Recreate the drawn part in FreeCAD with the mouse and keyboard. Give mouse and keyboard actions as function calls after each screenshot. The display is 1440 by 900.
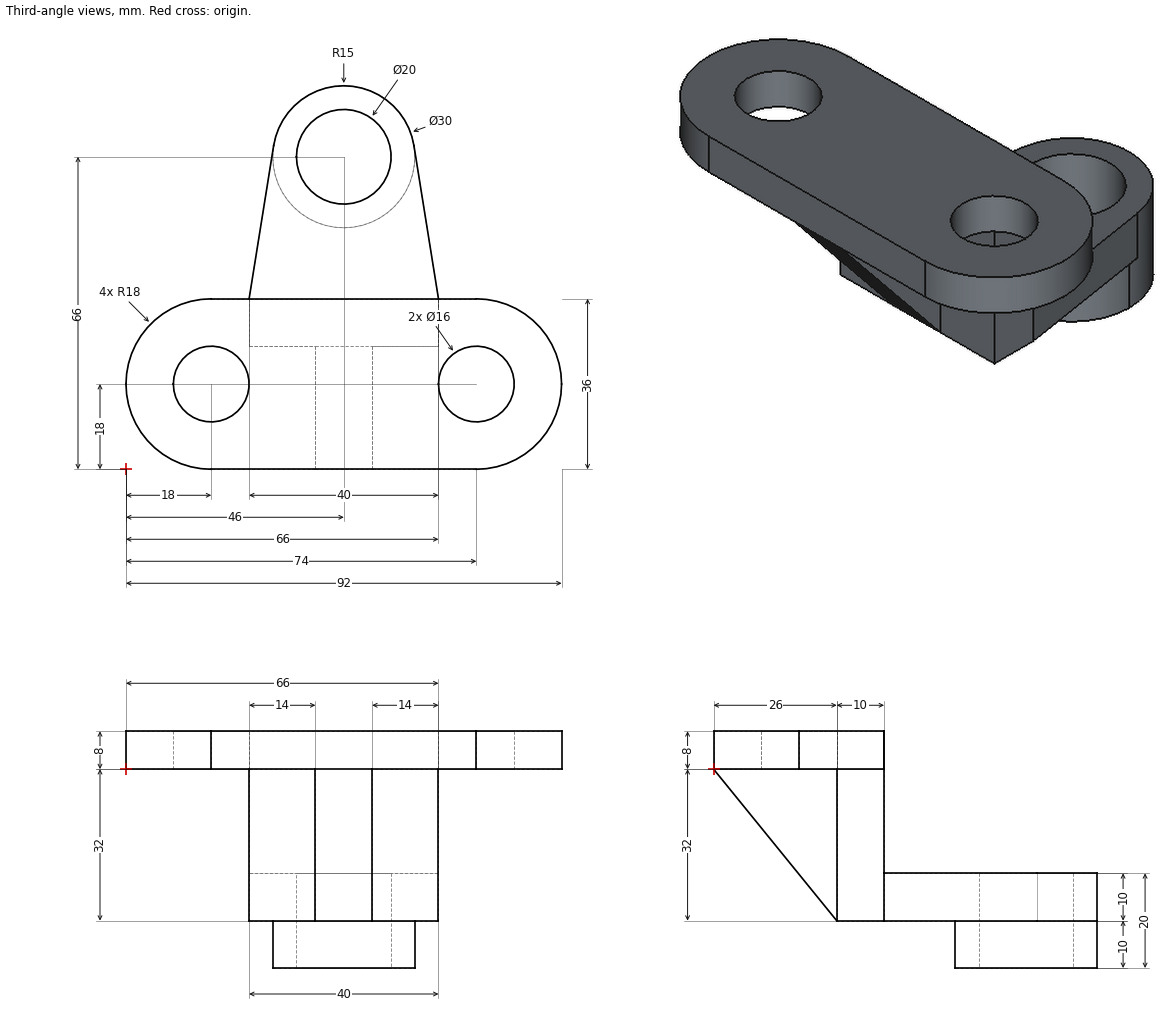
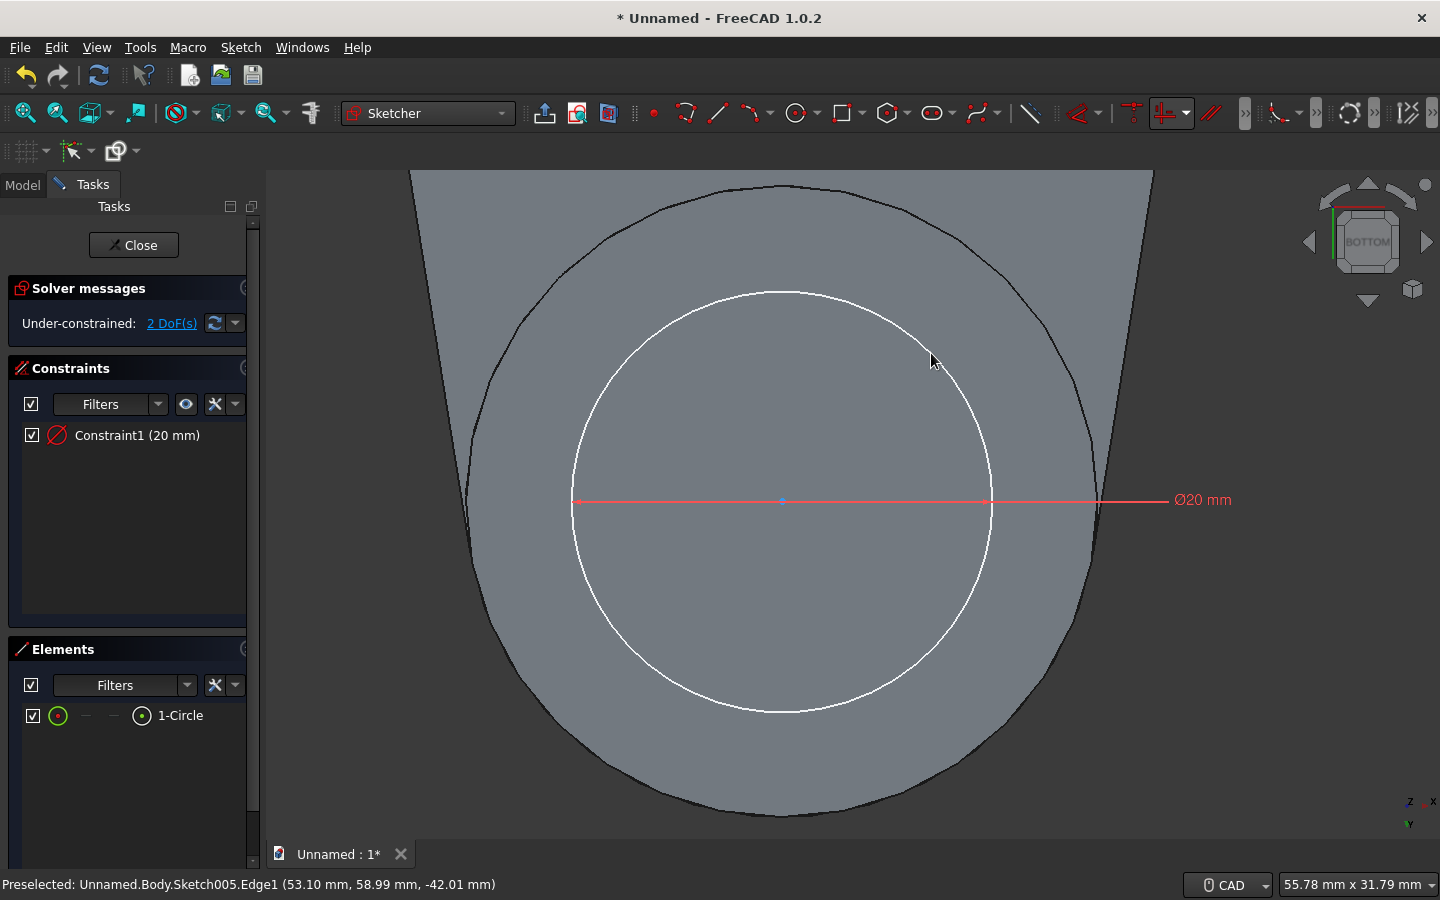
click(1078, 114)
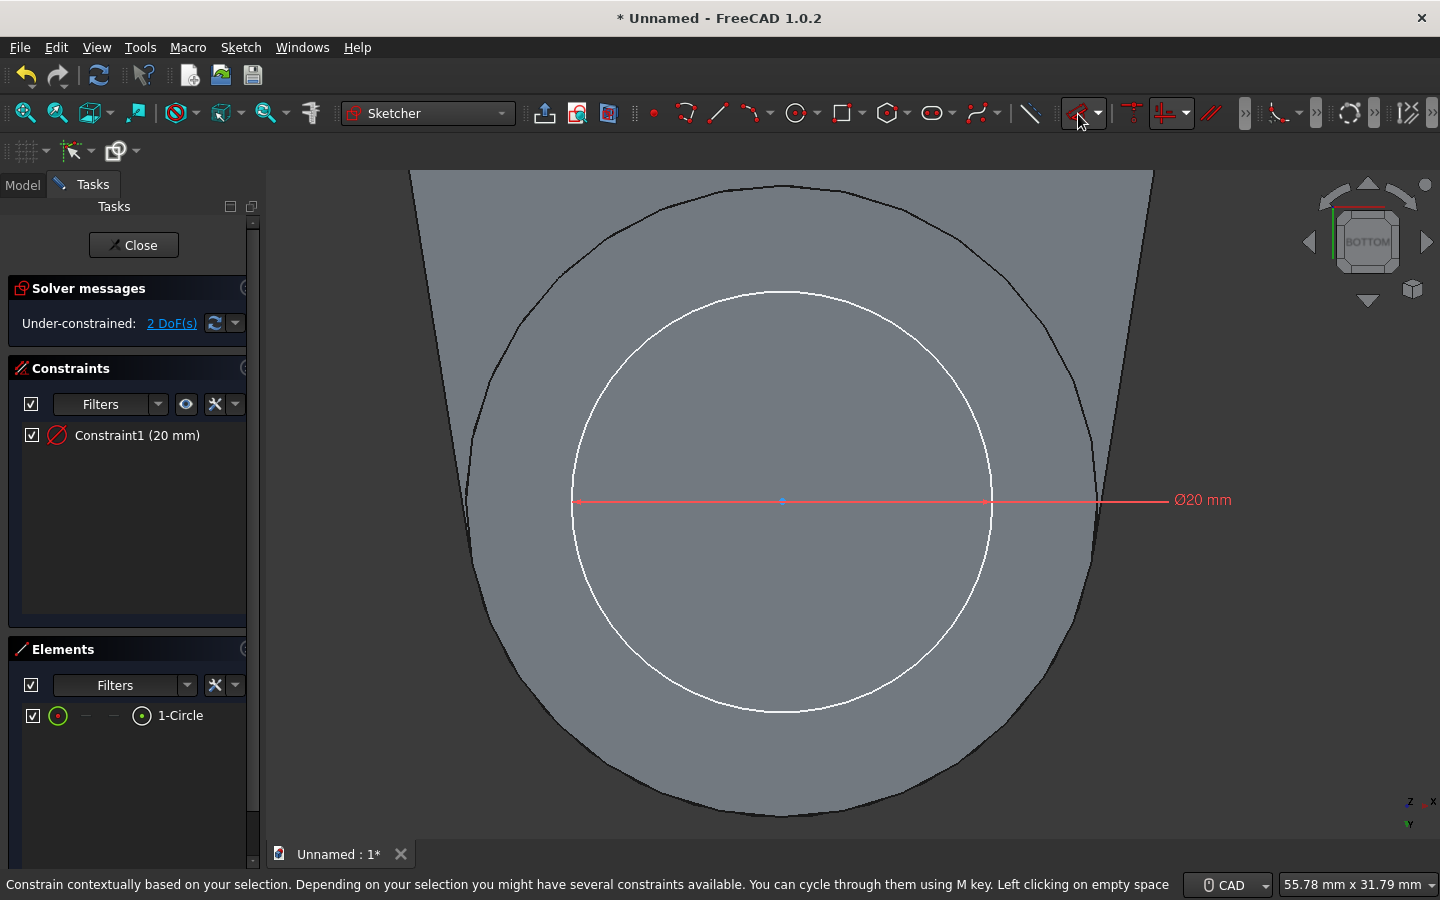
click(782, 502)
click(538, 536)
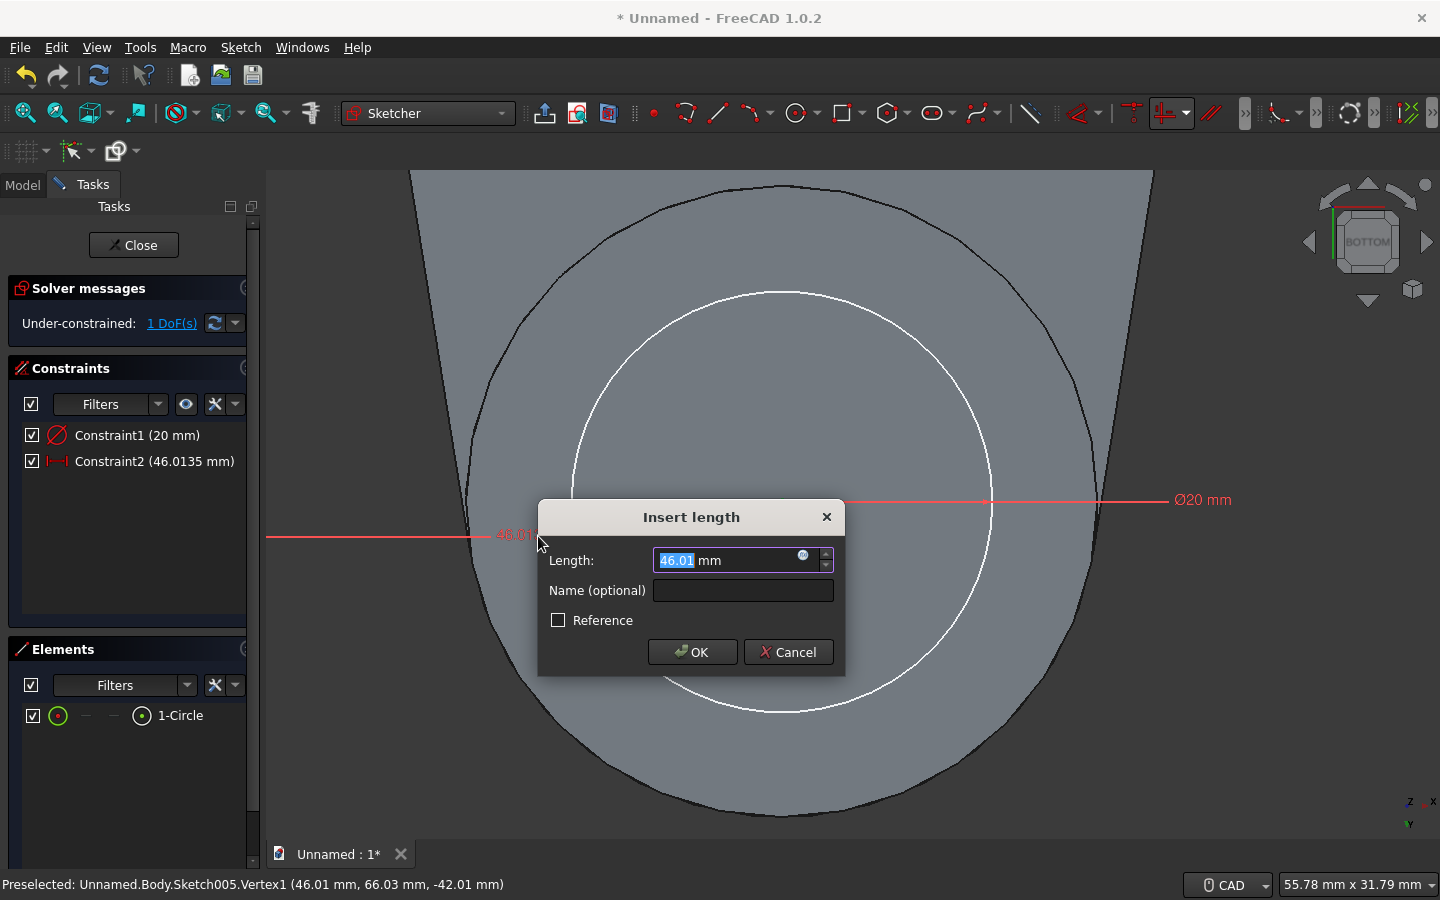
text(46)
key(Return)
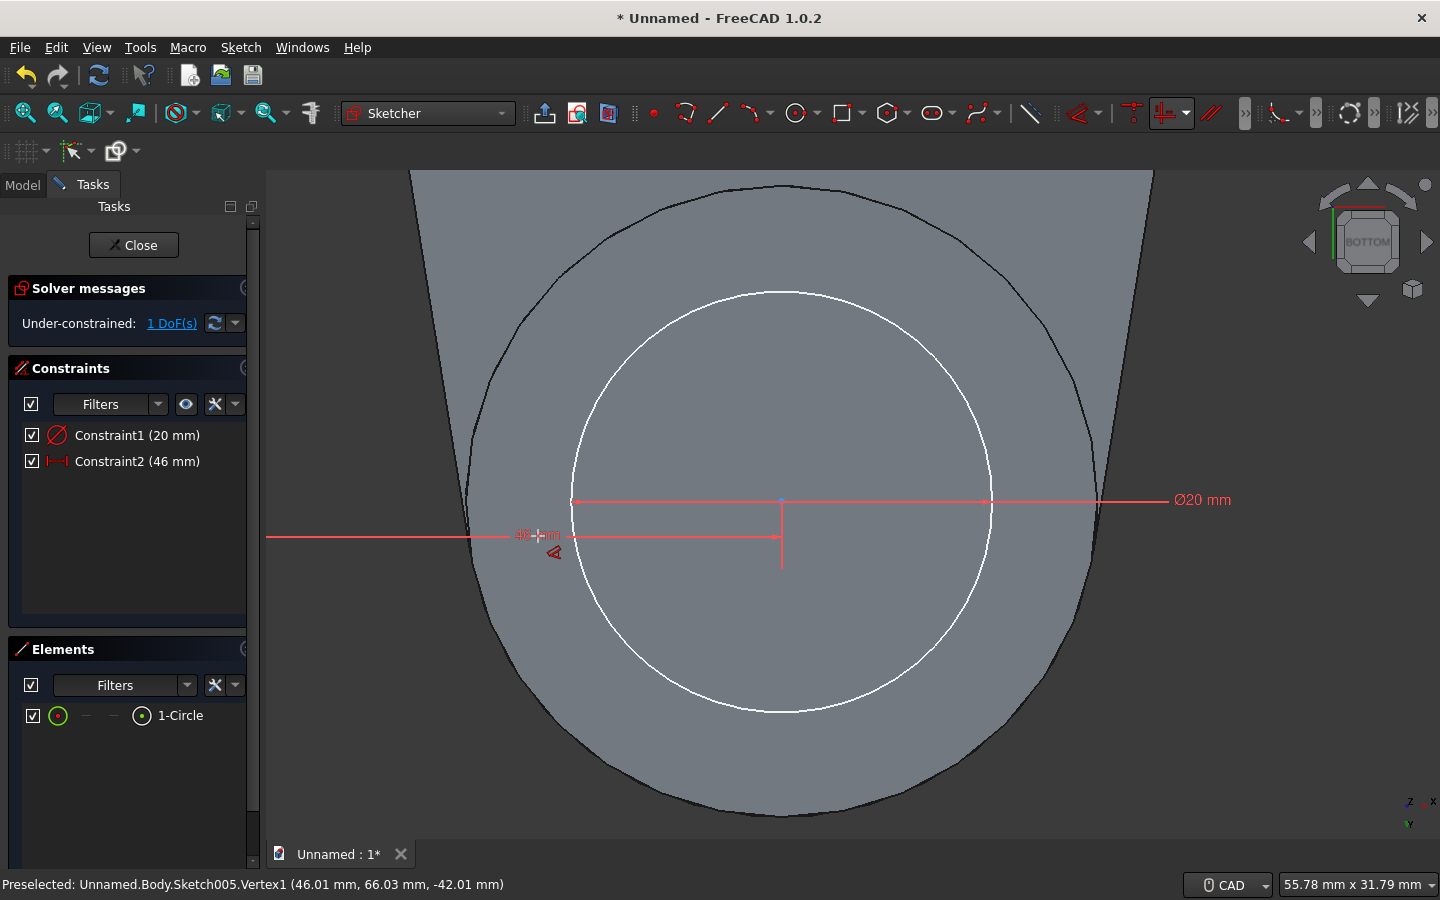
click(782, 502)
click(816, 350)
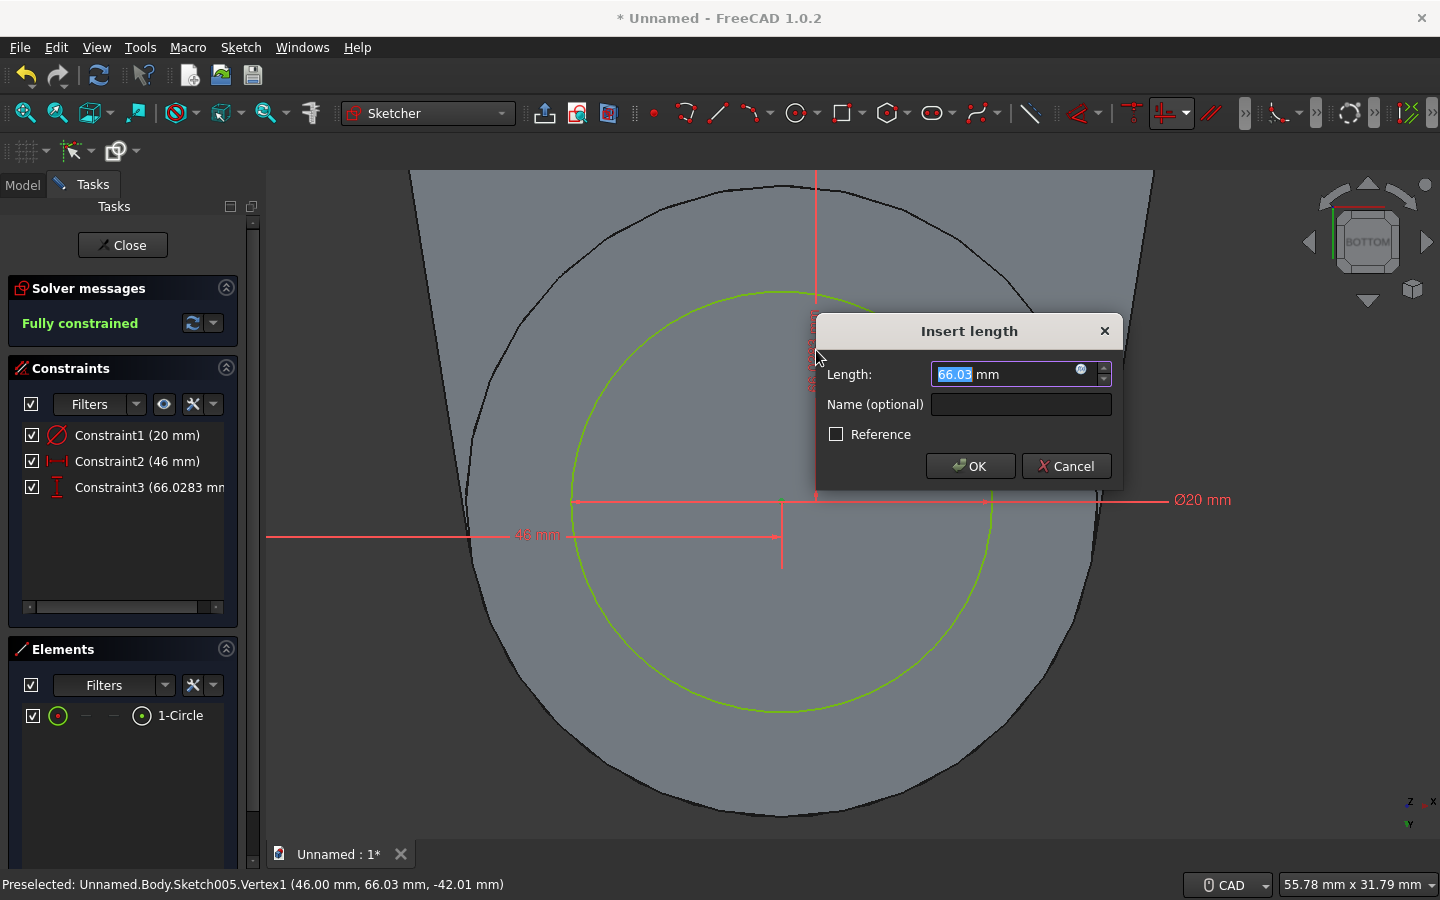
text(66)
key(Return)
key(Escape)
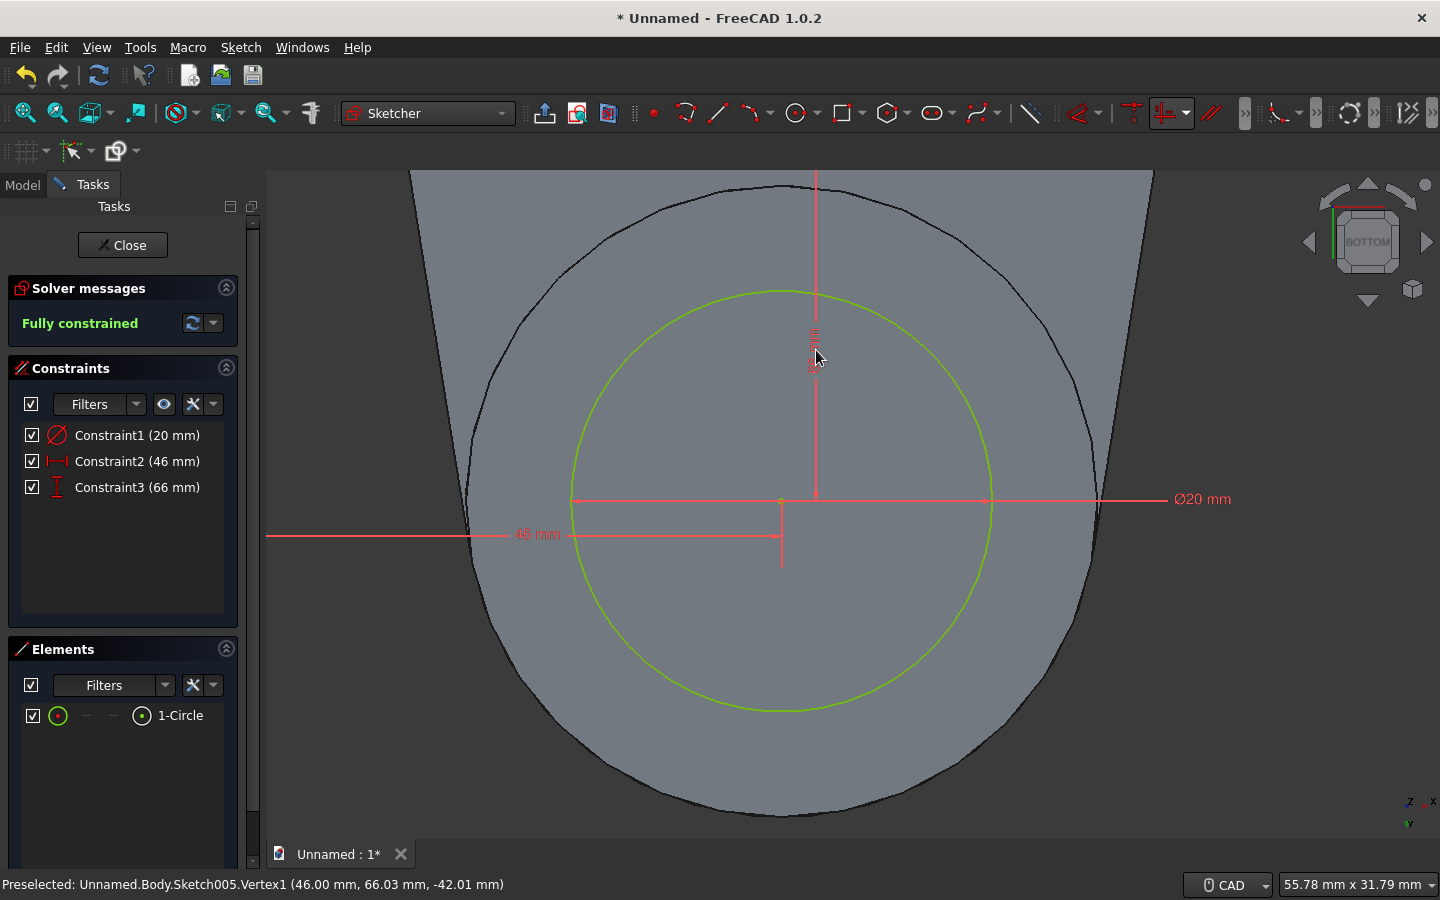
click(123, 245)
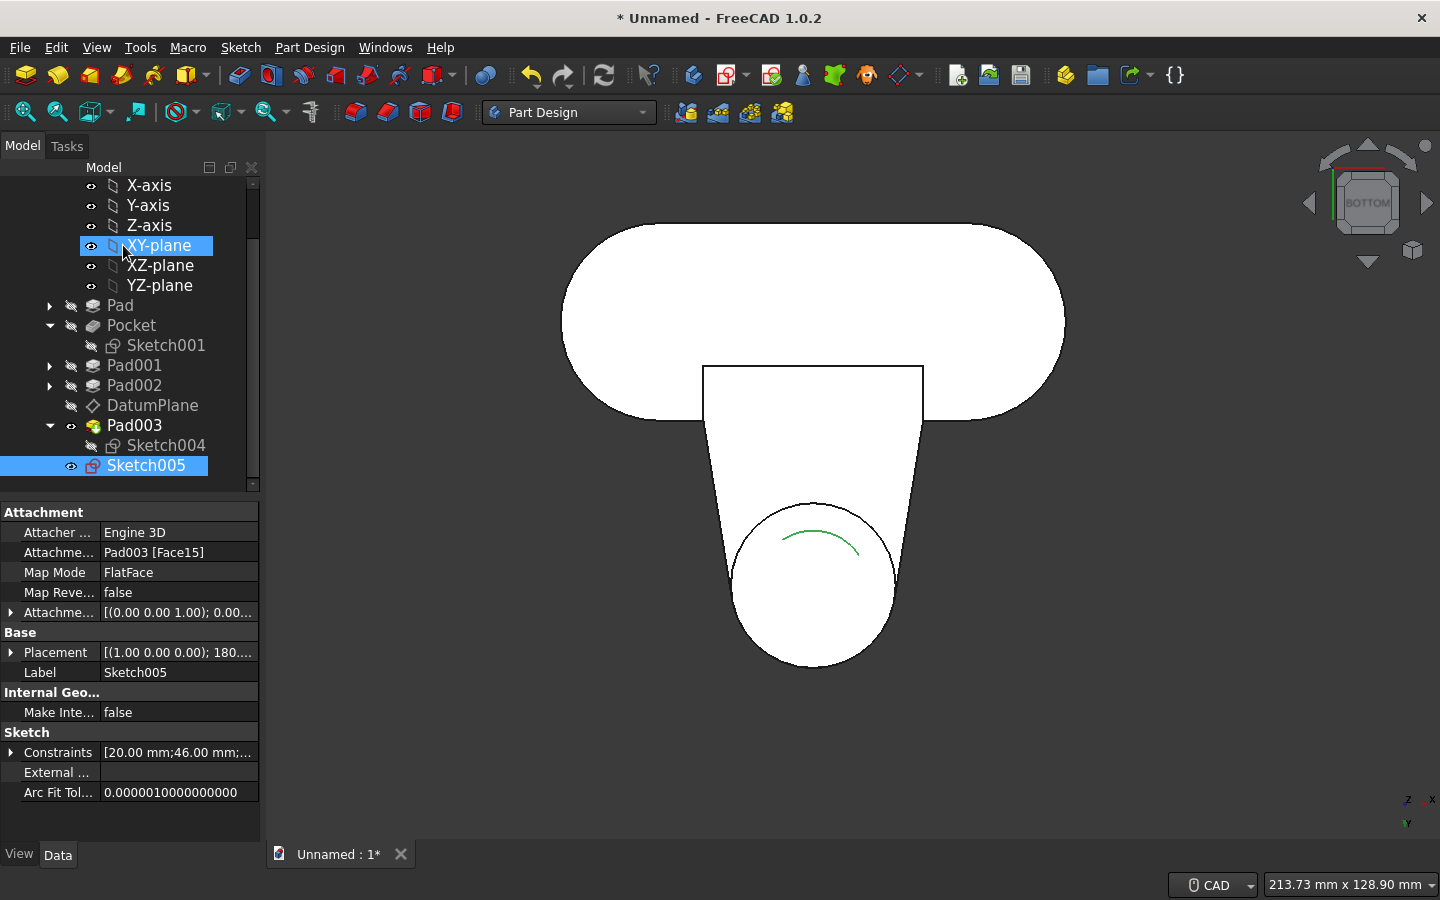
click(240, 76)